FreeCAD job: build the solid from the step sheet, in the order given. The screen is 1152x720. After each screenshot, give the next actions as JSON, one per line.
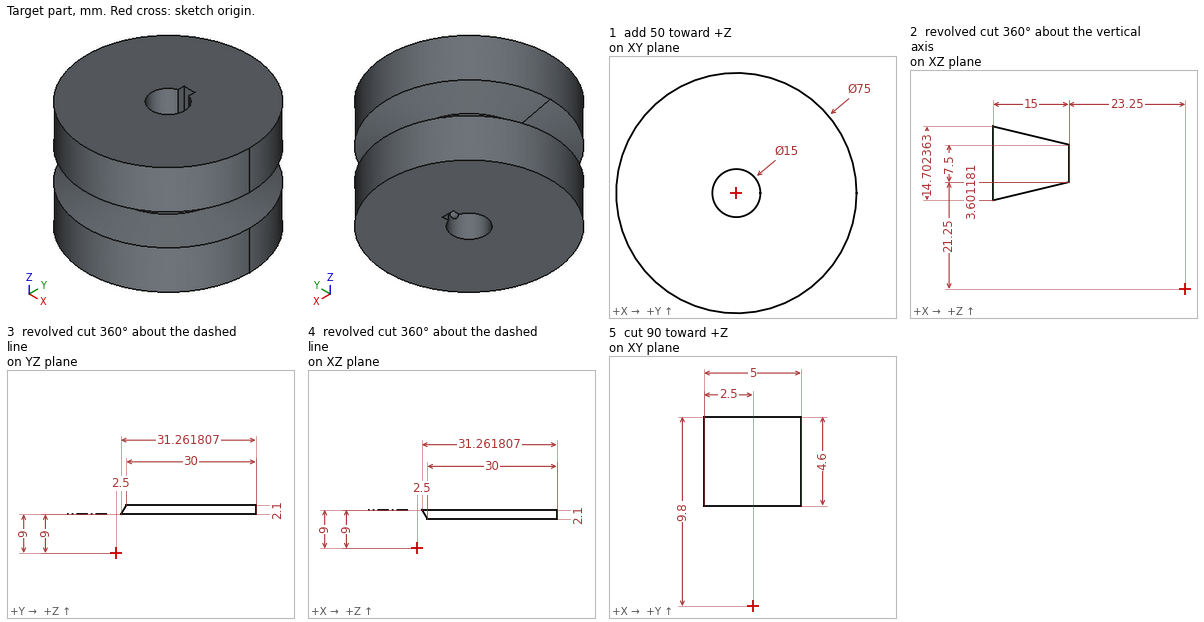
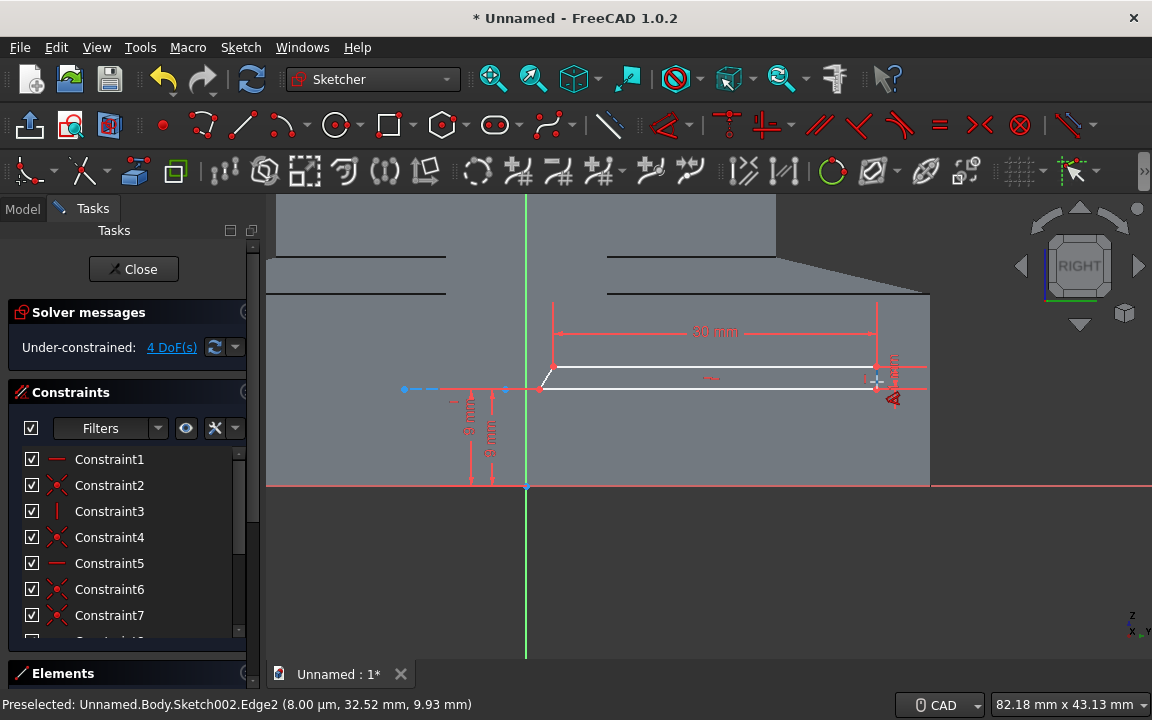
{"action": "scroll", "coordinate": [553, 367], "scroll_direction": "up", "scroll_amount": 2}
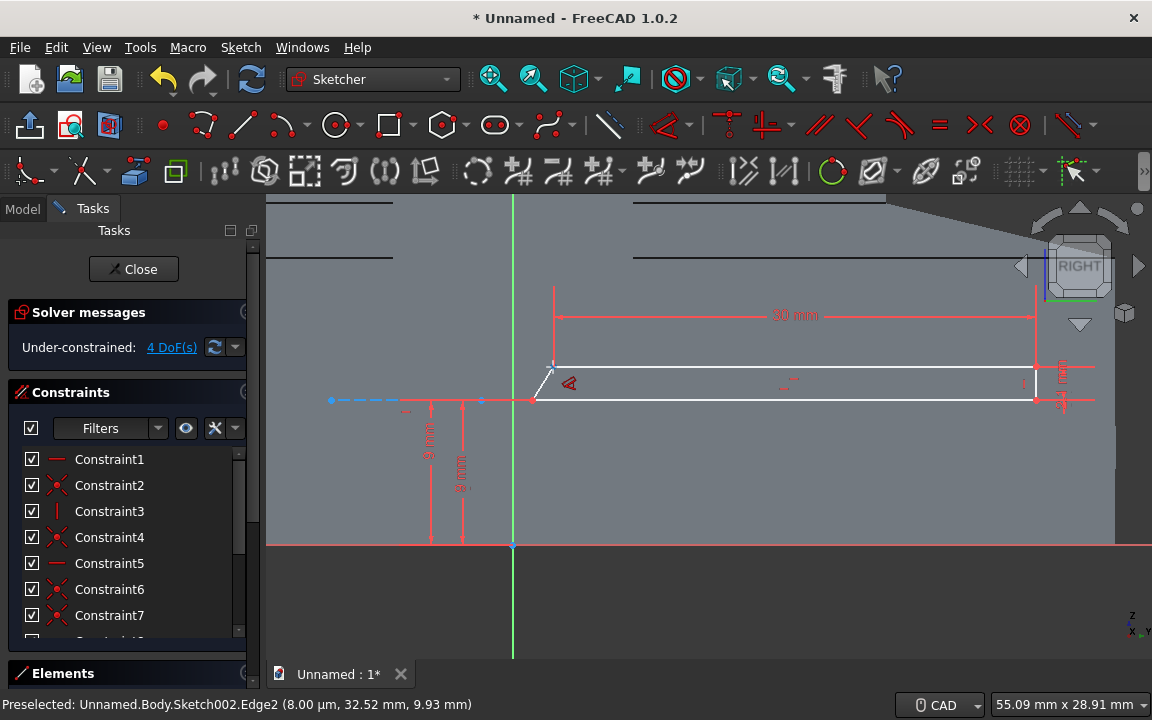
{"action": "left_click", "coordinate": [554, 367]}
{"action": "left_click", "coordinate": [533, 579]}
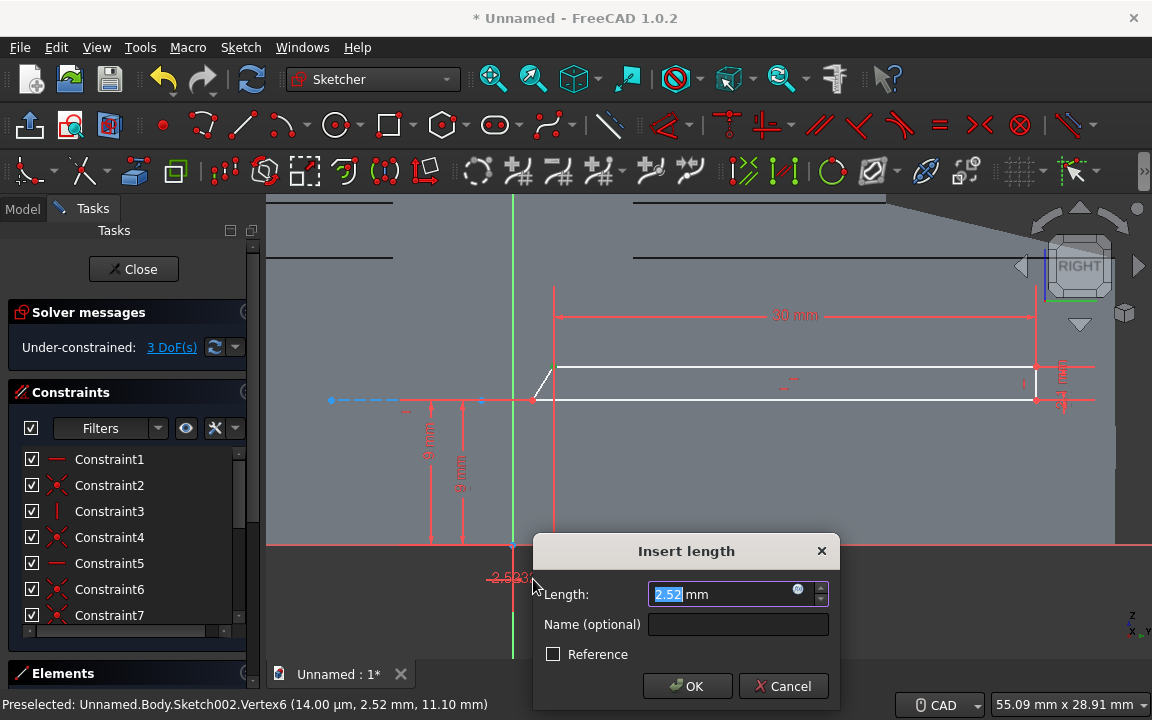
{"action": "type", "text": "2.5"}
{"action": "key", "text": "Return"}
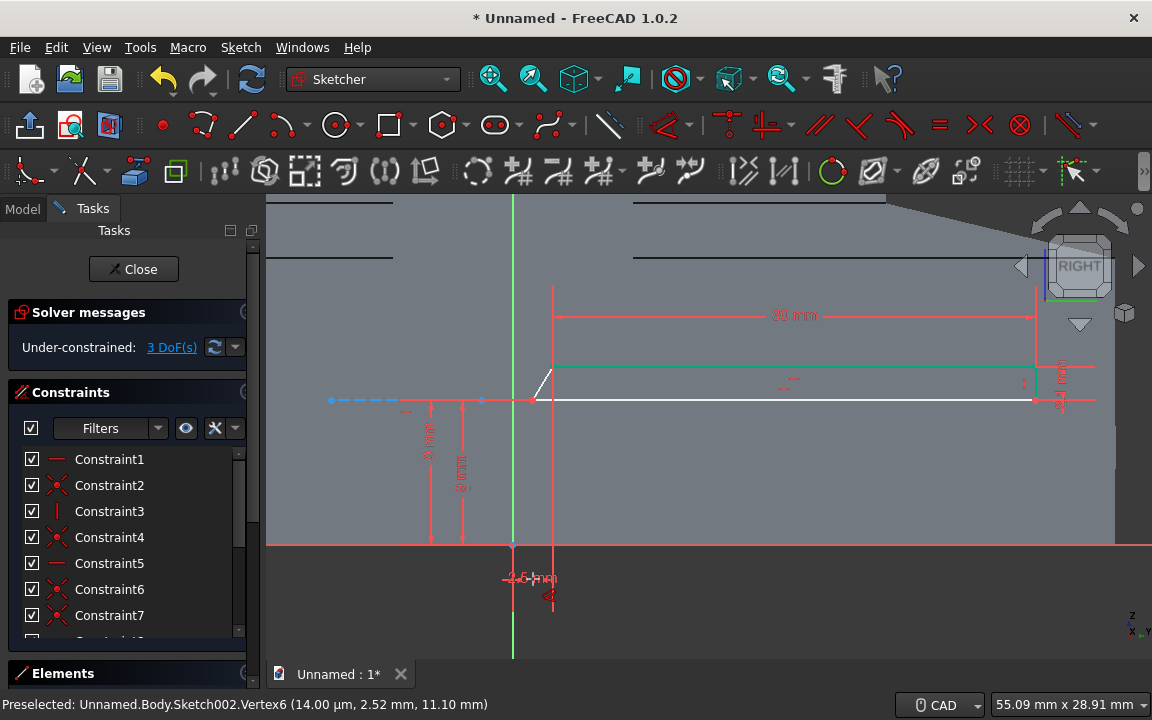
{"action": "left_click", "coordinate": [684, 400]}
{"action": "left_click", "coordinate": [760, 434]}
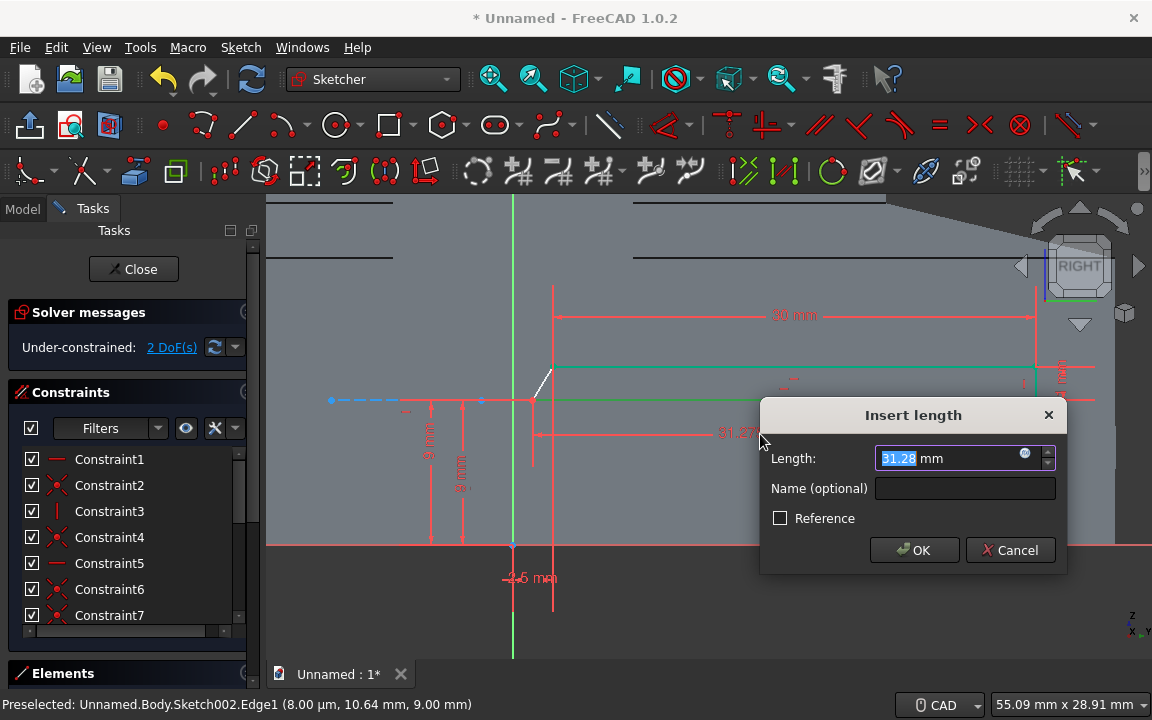
{"action": "type", "text": "31.261807"}
{"action": "key", "text": "Return"}
{"action": "key", "text": "Escape"}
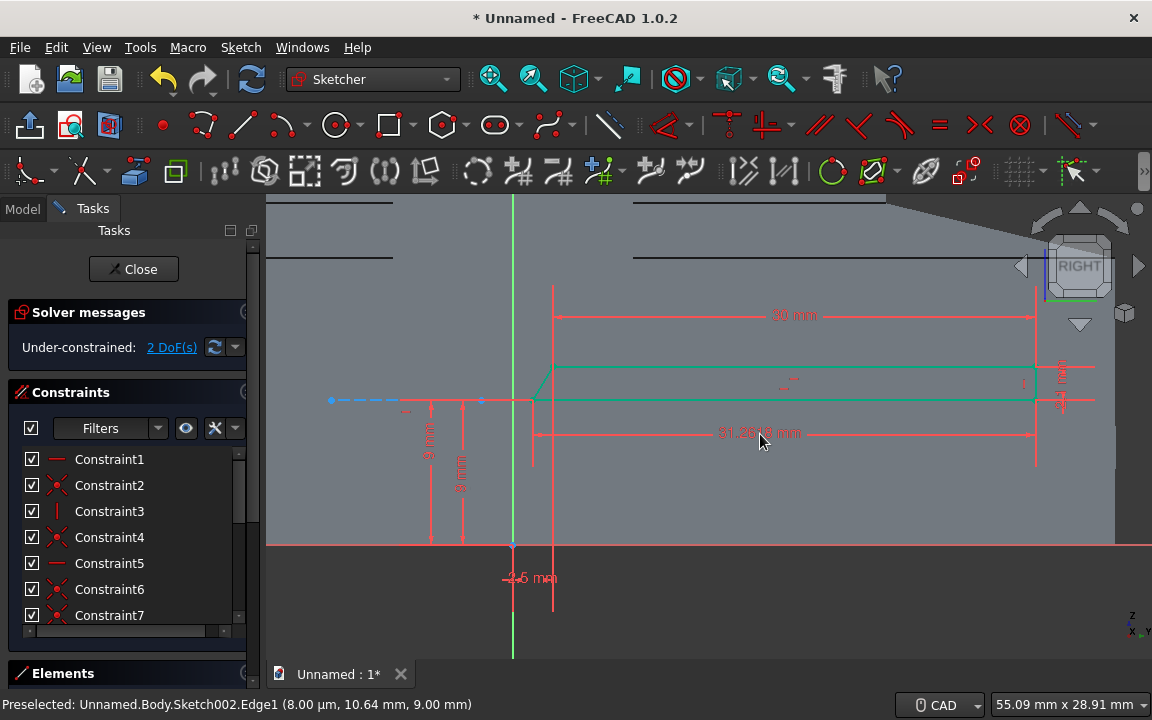
{"action": "left_click", "coordinate": [134, 269]}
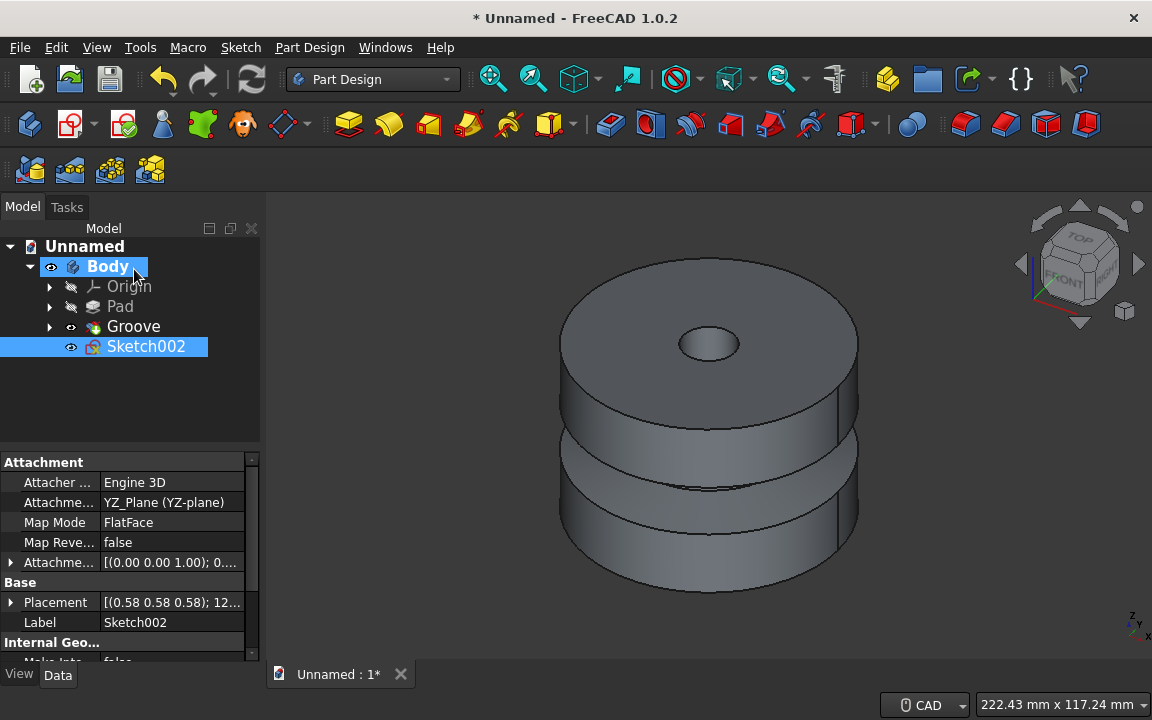
{"action": "left_click", "coordinate": [692, 124]}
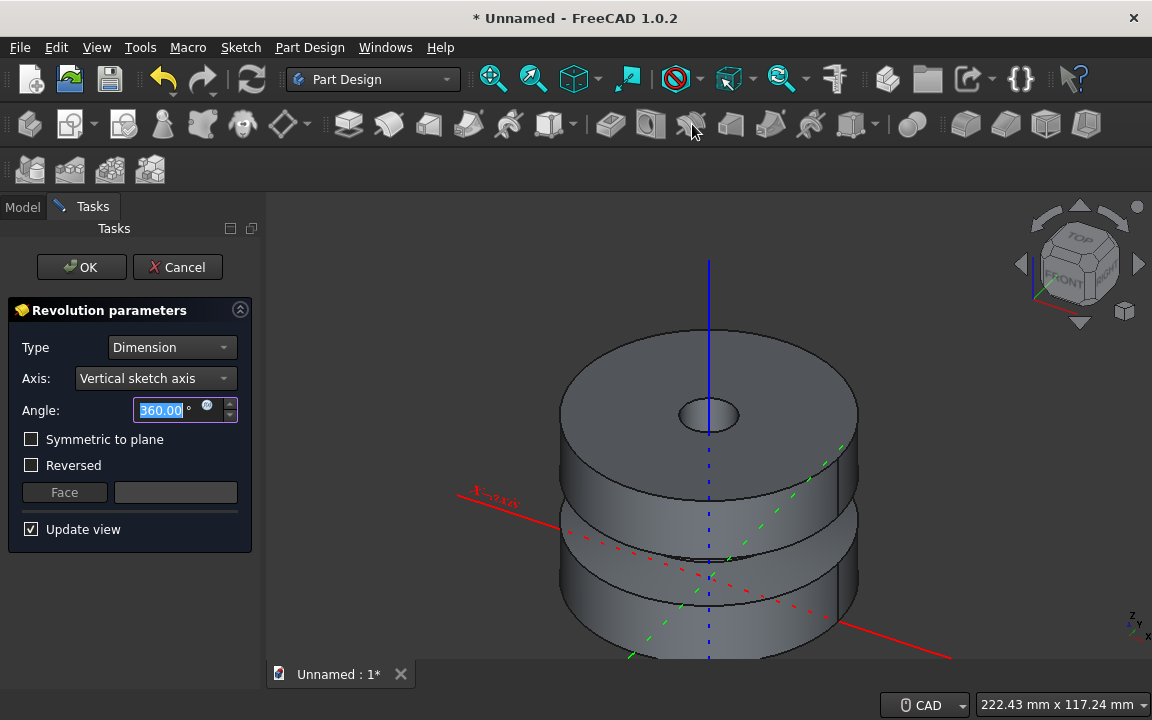
{"action": "left_click", "coordinate": [156, 378]}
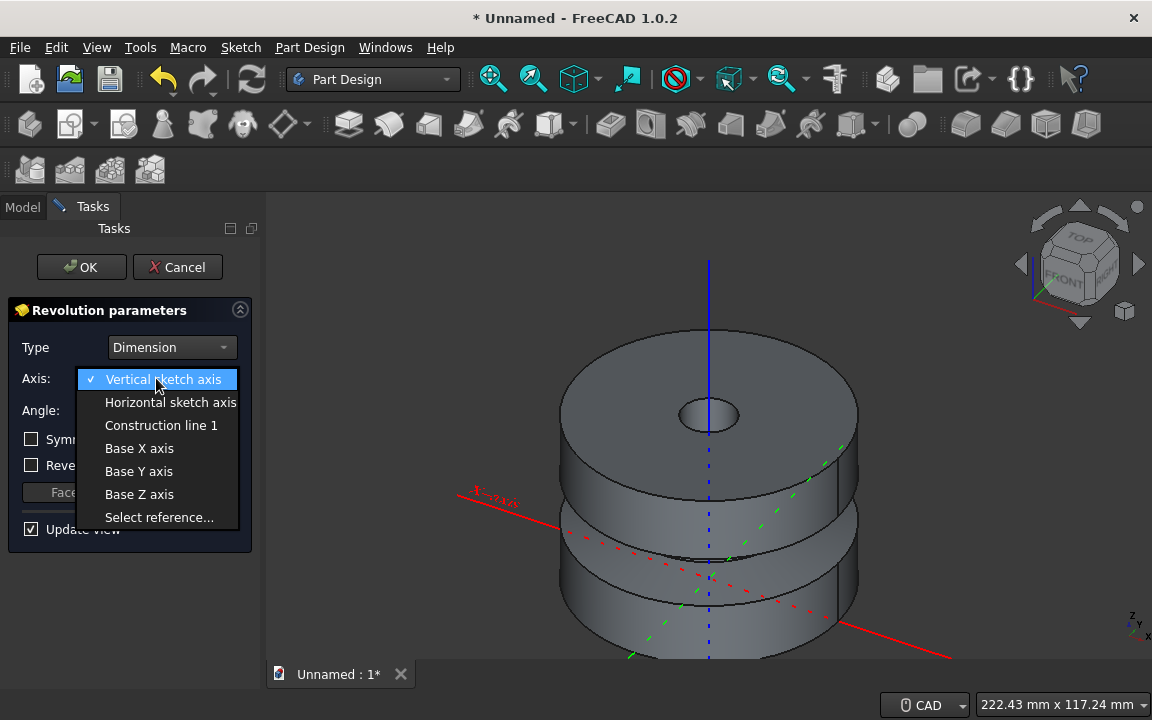
{"action": "left_click", "coordinate": [156, 426]}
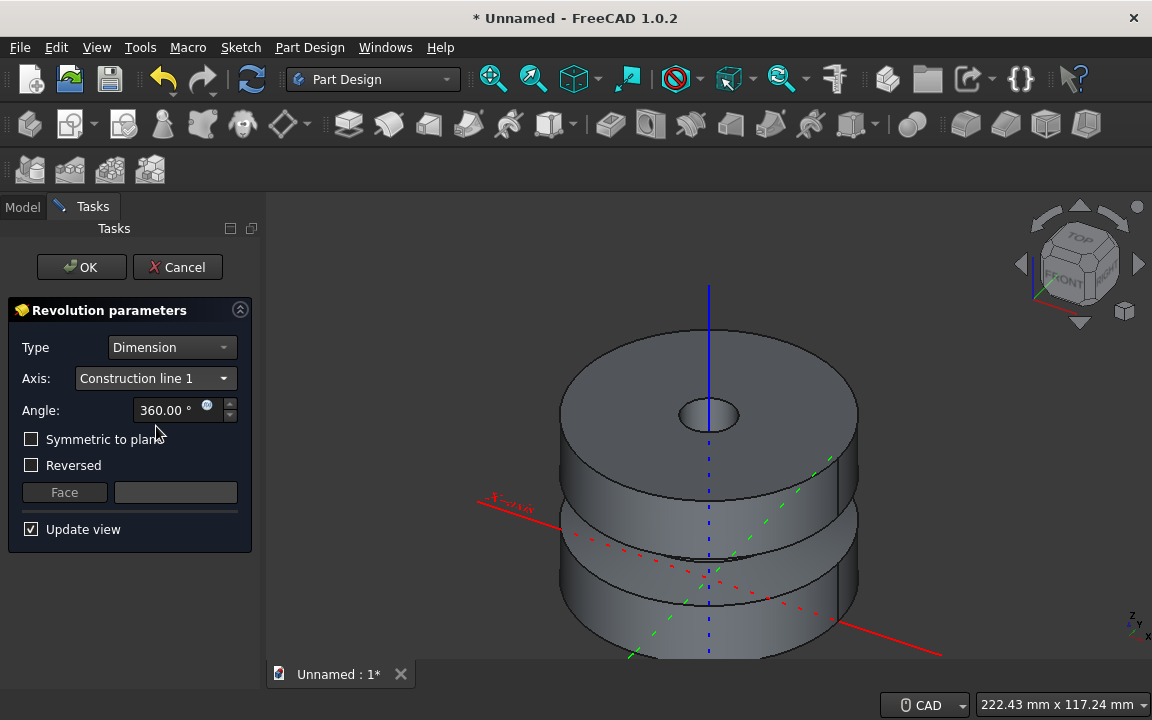
{"action": "left_click", "coordinate": [82, 267]}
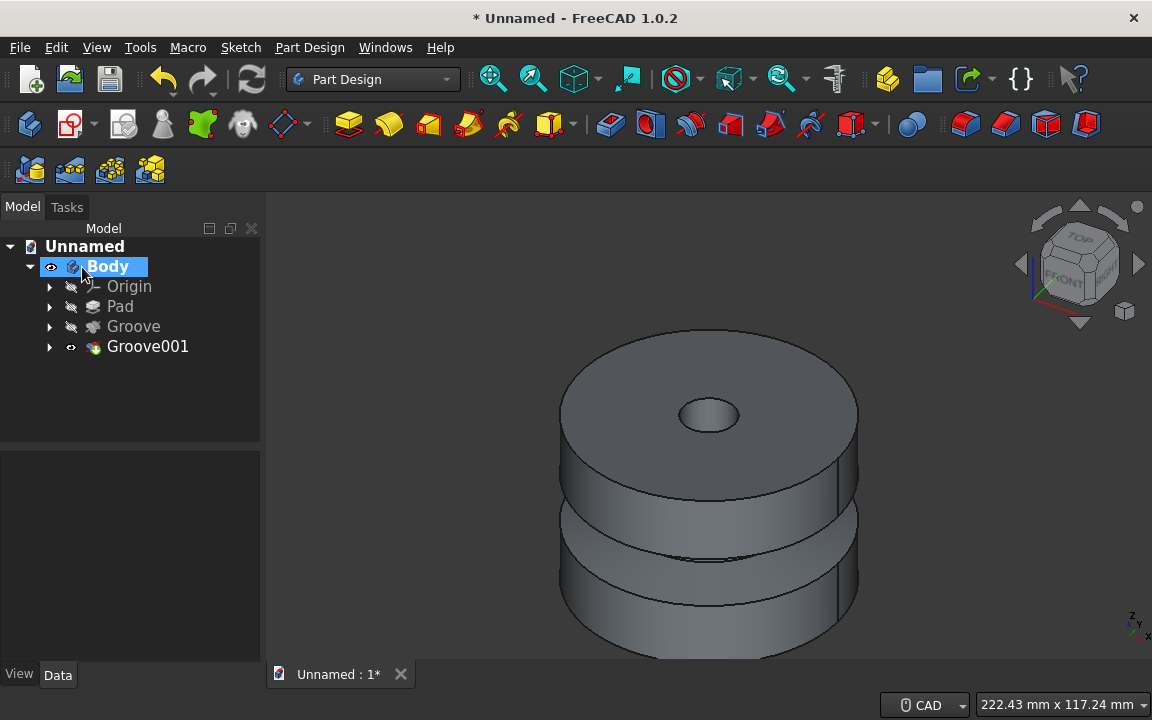
{"action": "left_click", "coordinate": [494, 80]}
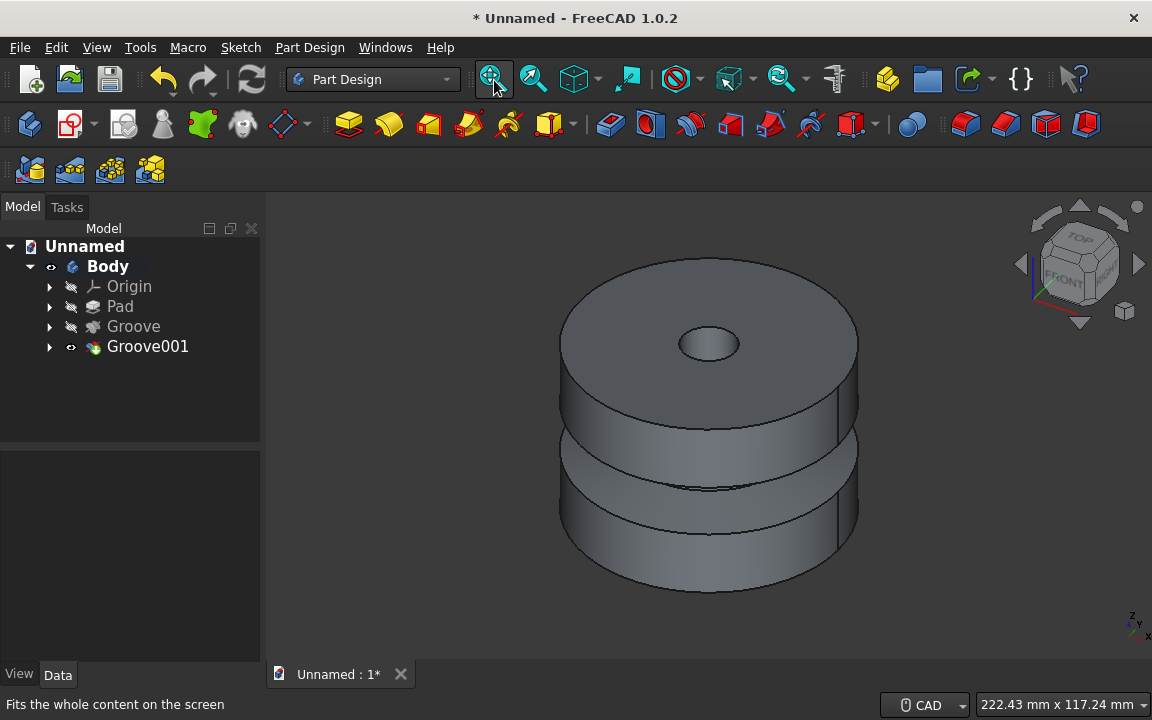
{"action": "left_click", "coordinate": [70, 124]}